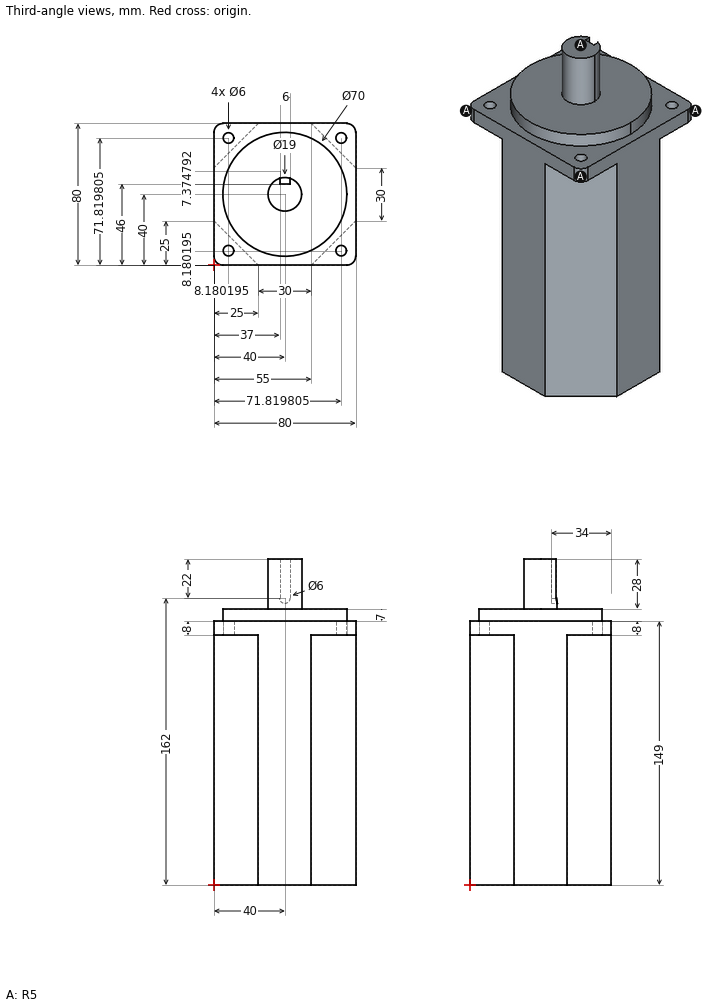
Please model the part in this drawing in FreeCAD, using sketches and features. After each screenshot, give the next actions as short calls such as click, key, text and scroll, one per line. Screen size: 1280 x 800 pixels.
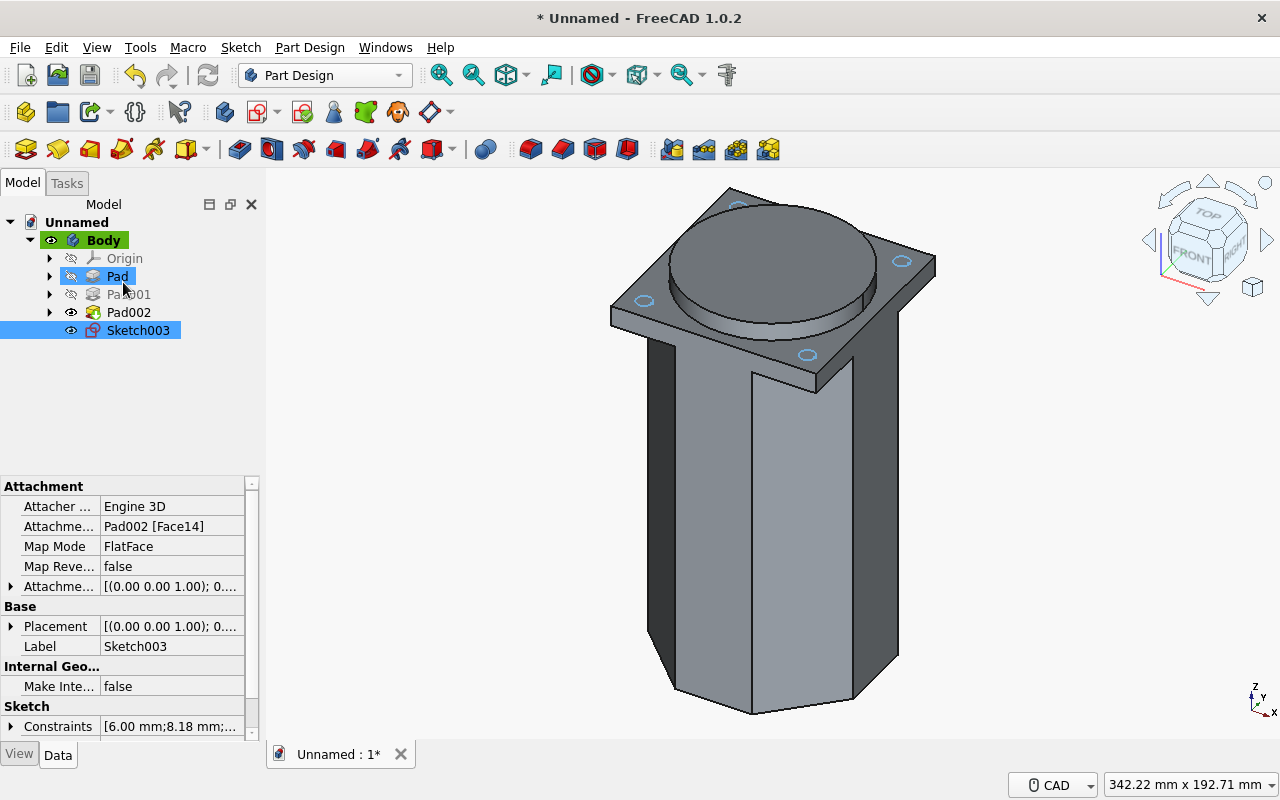
click(240, 150)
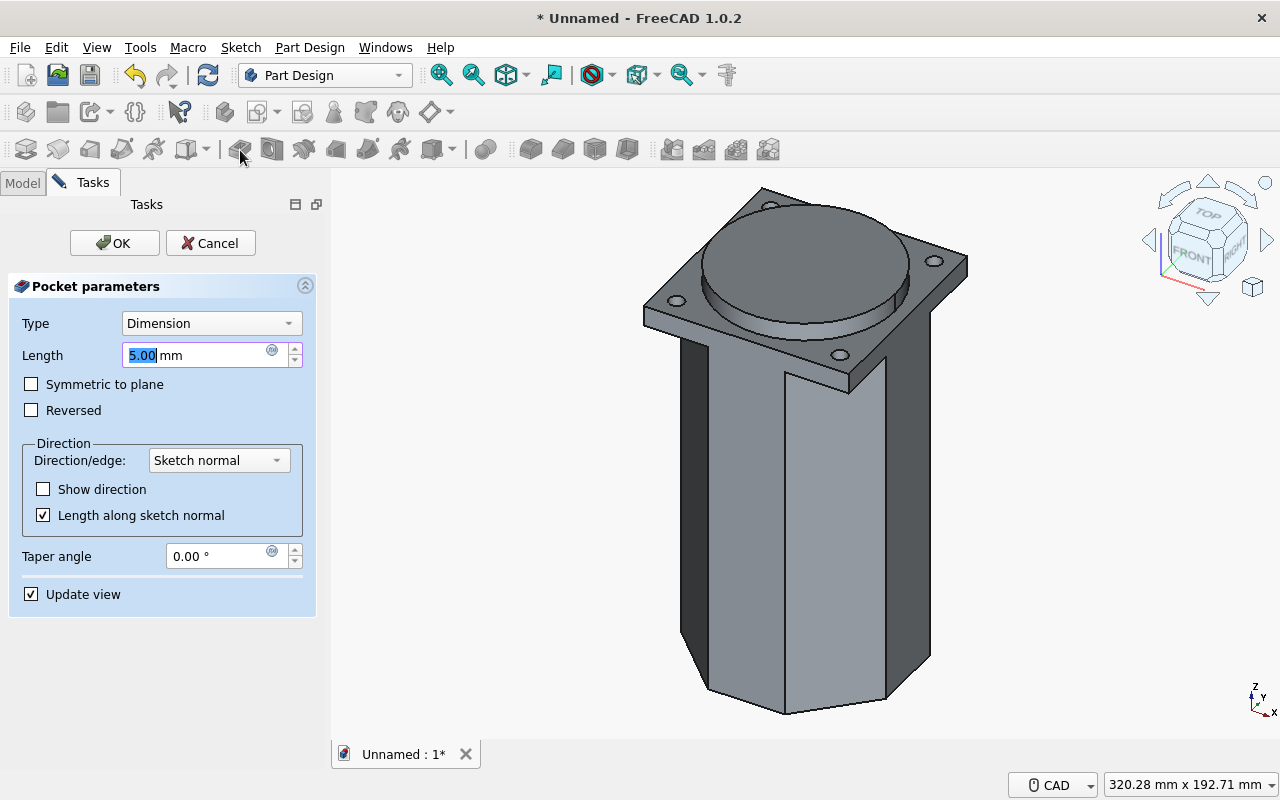
text(8)
key(Tab)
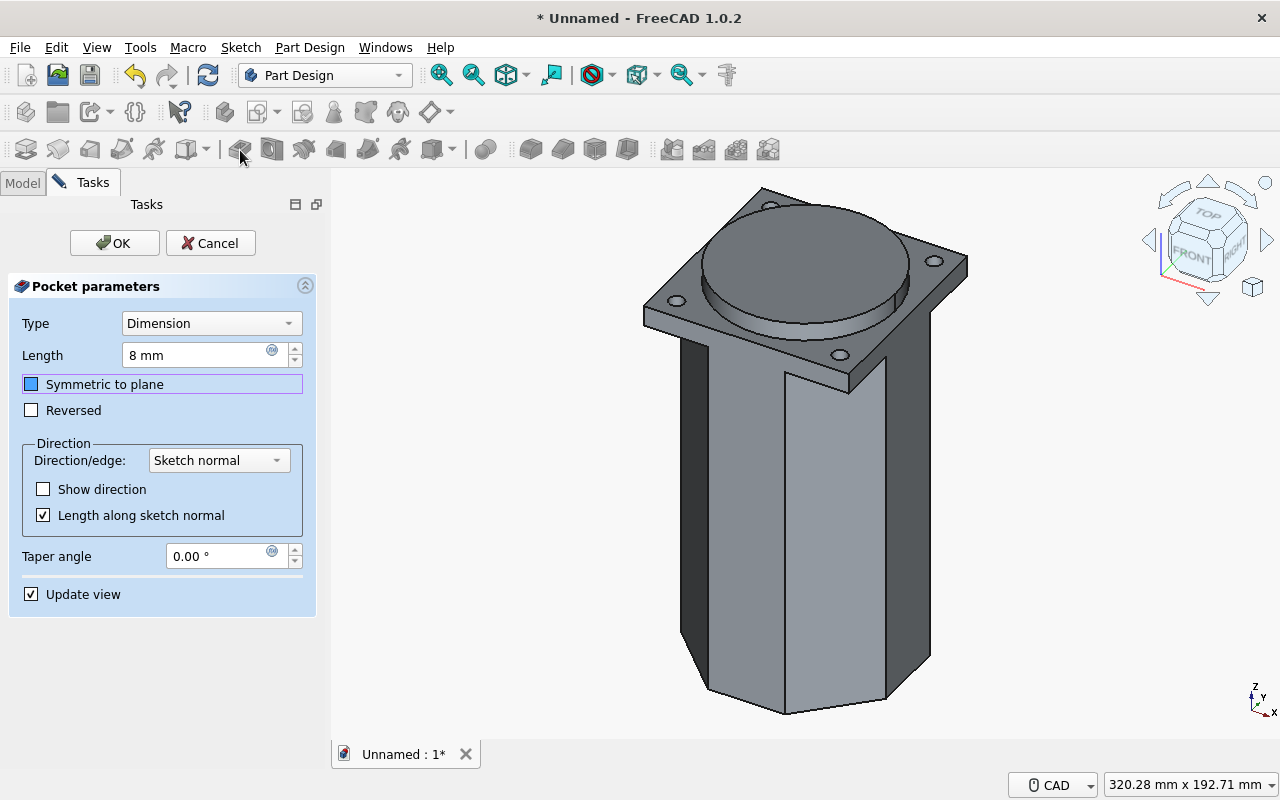
click(115, 243)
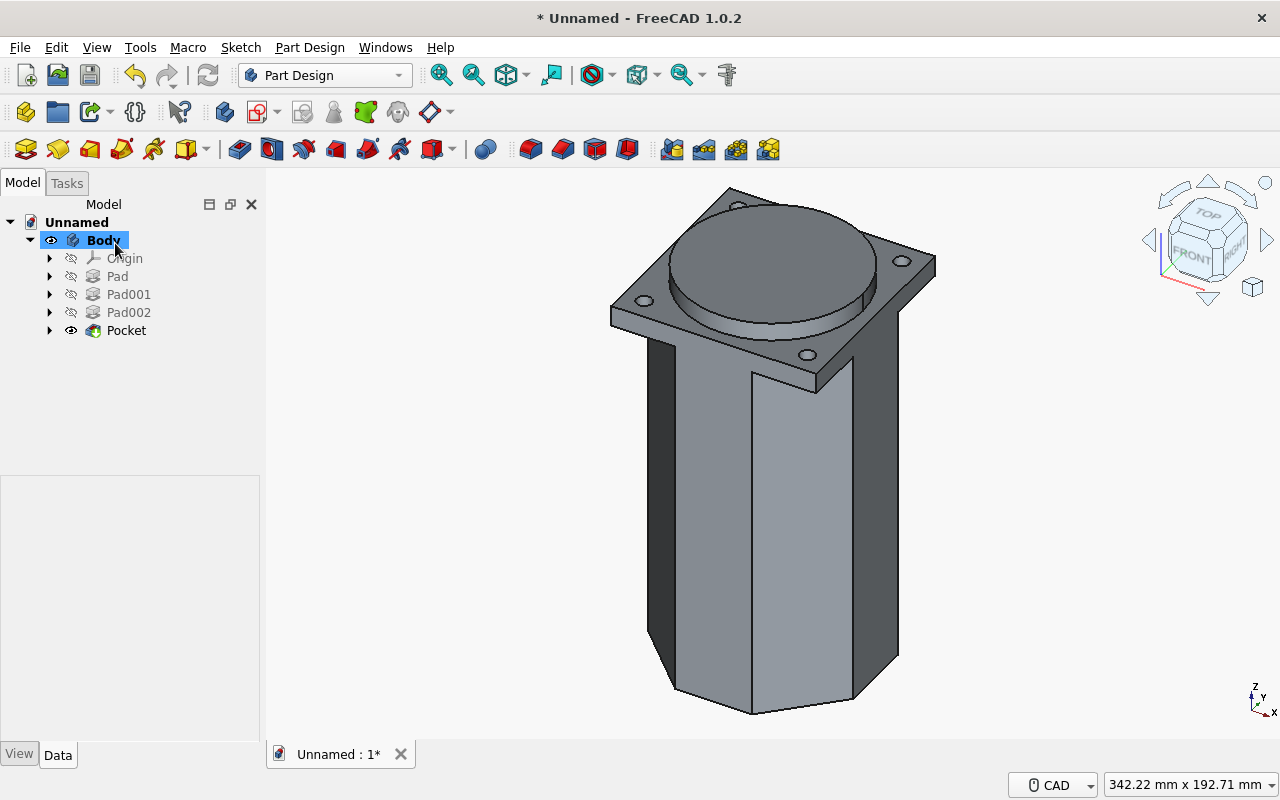
click(816, 383)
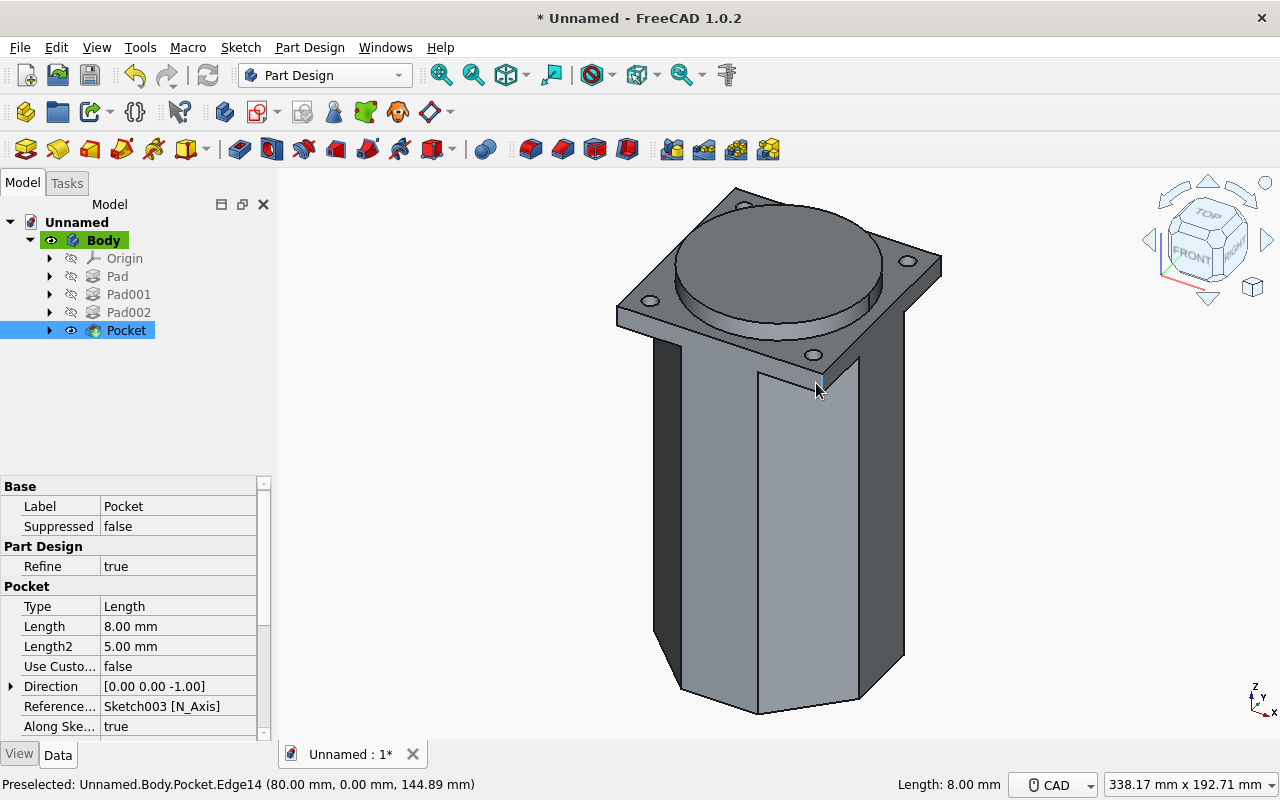
key(0)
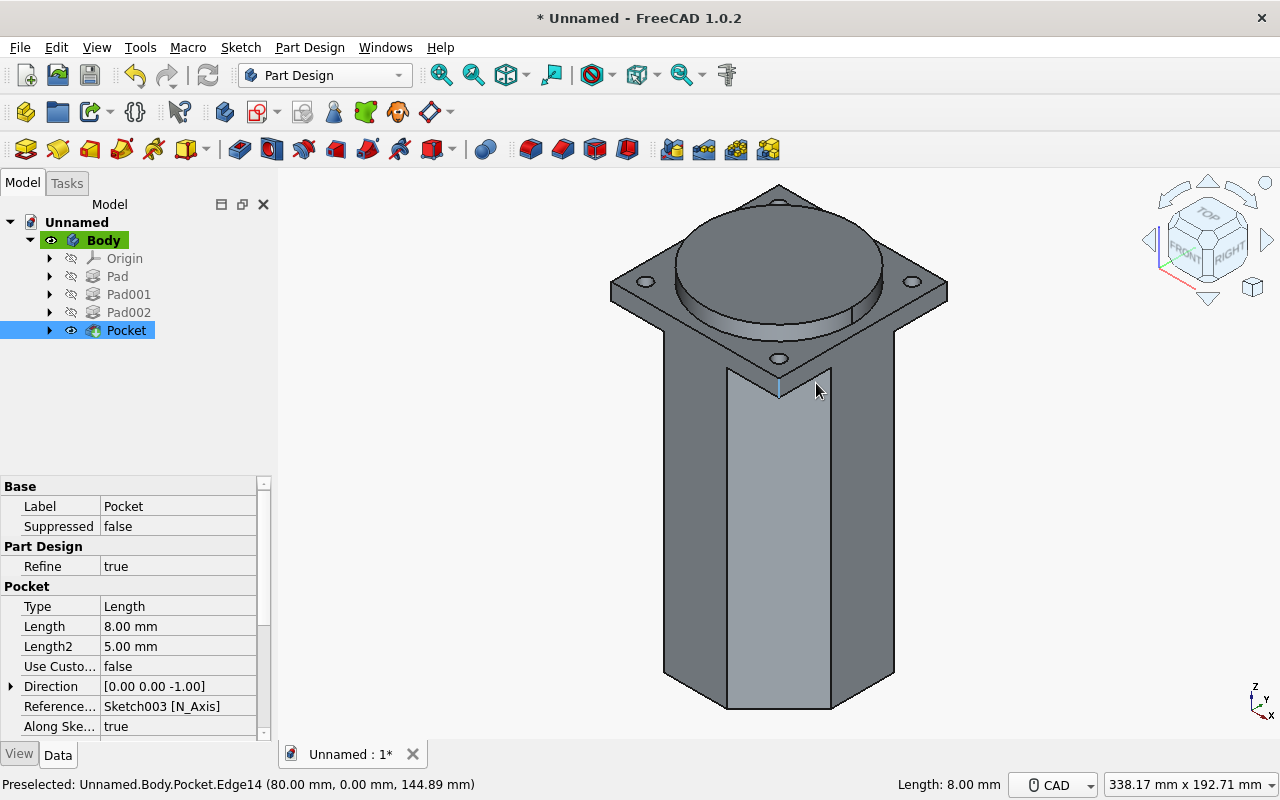
key(v)
key(f)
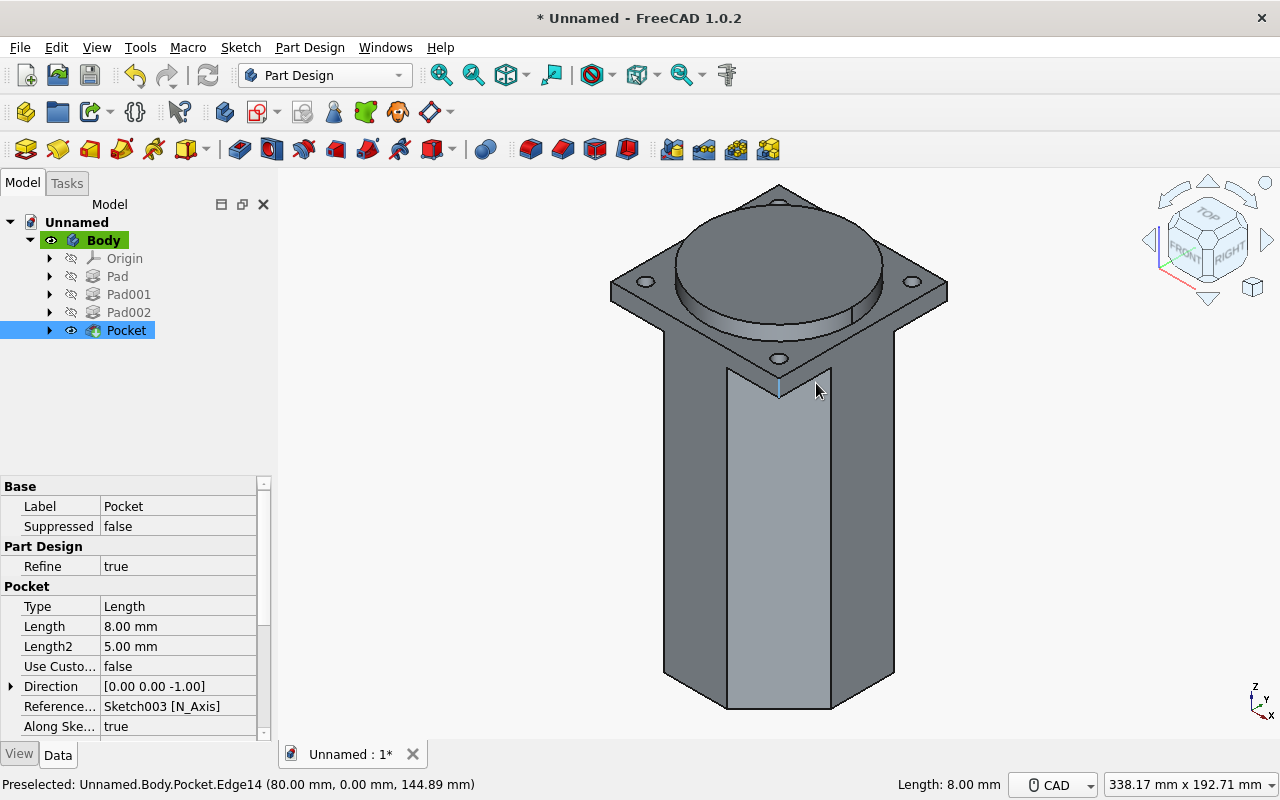
key(2)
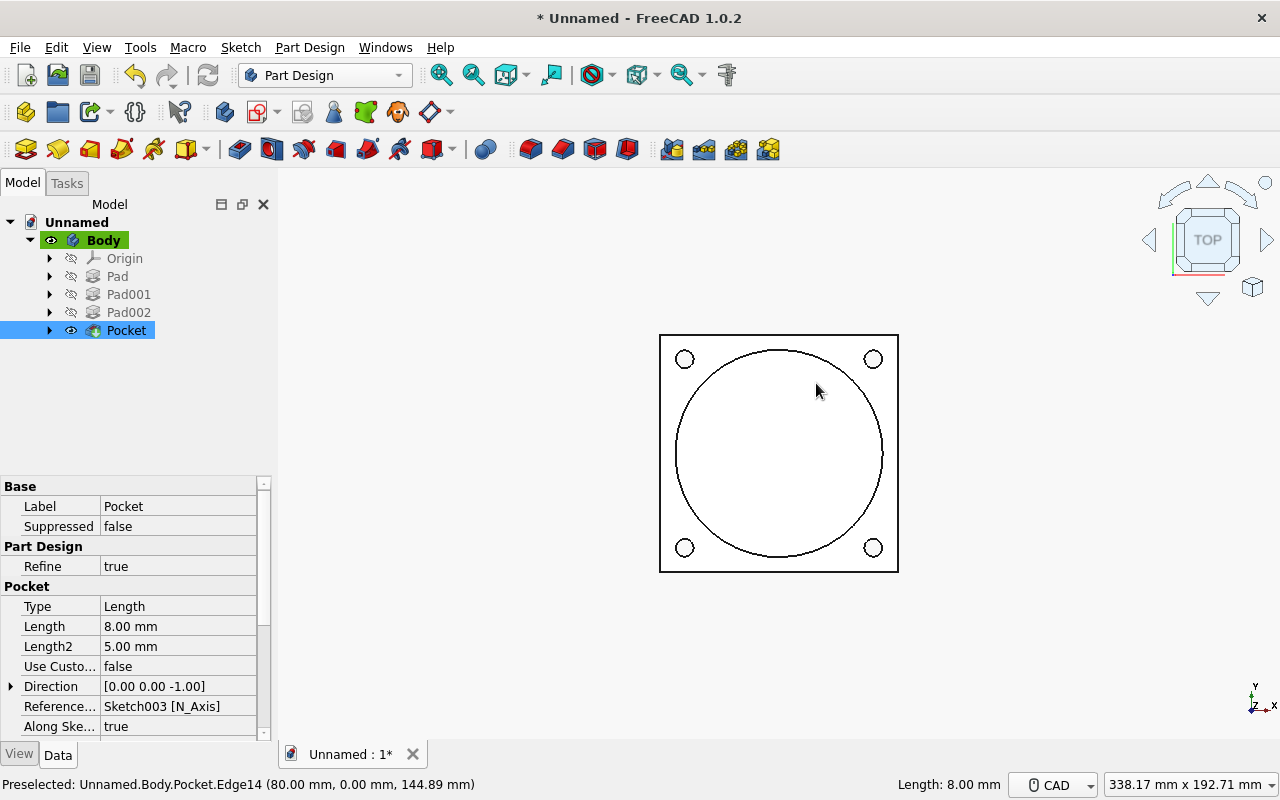
key(v)
key(f)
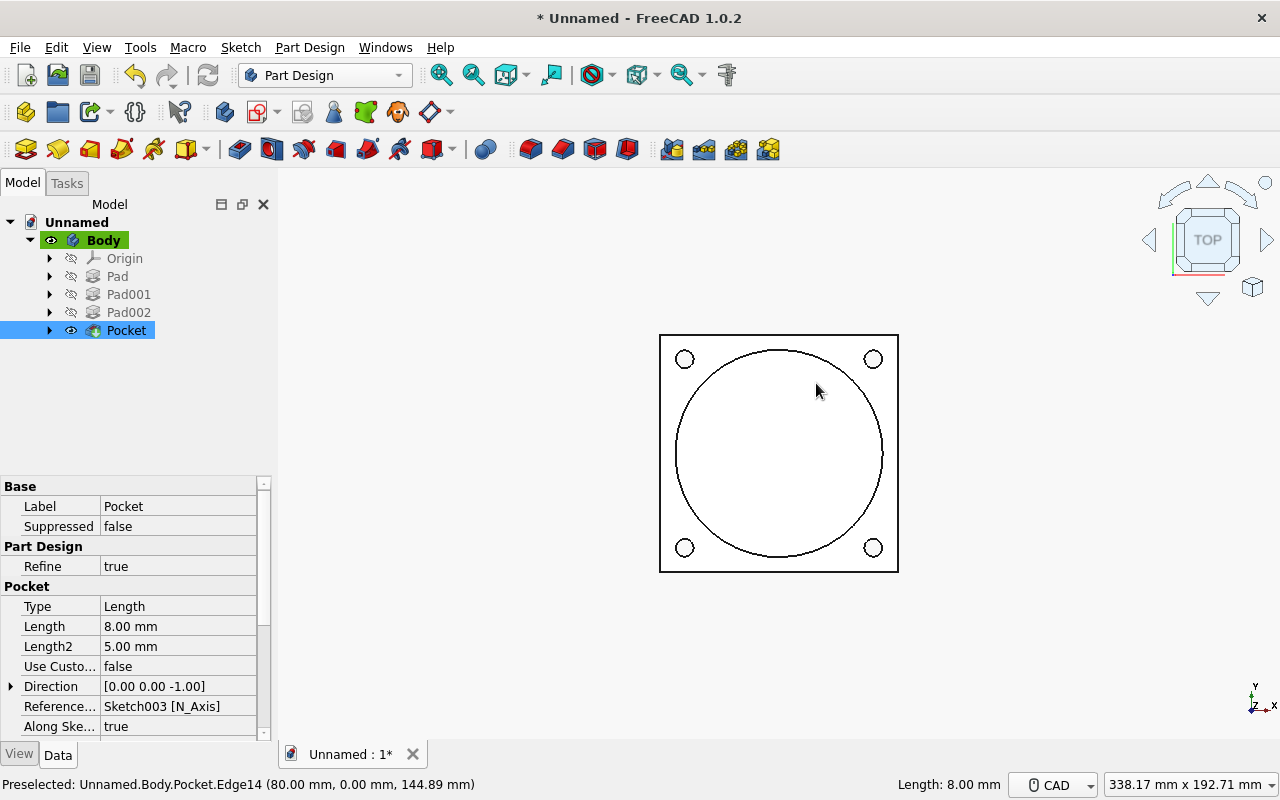
key(1)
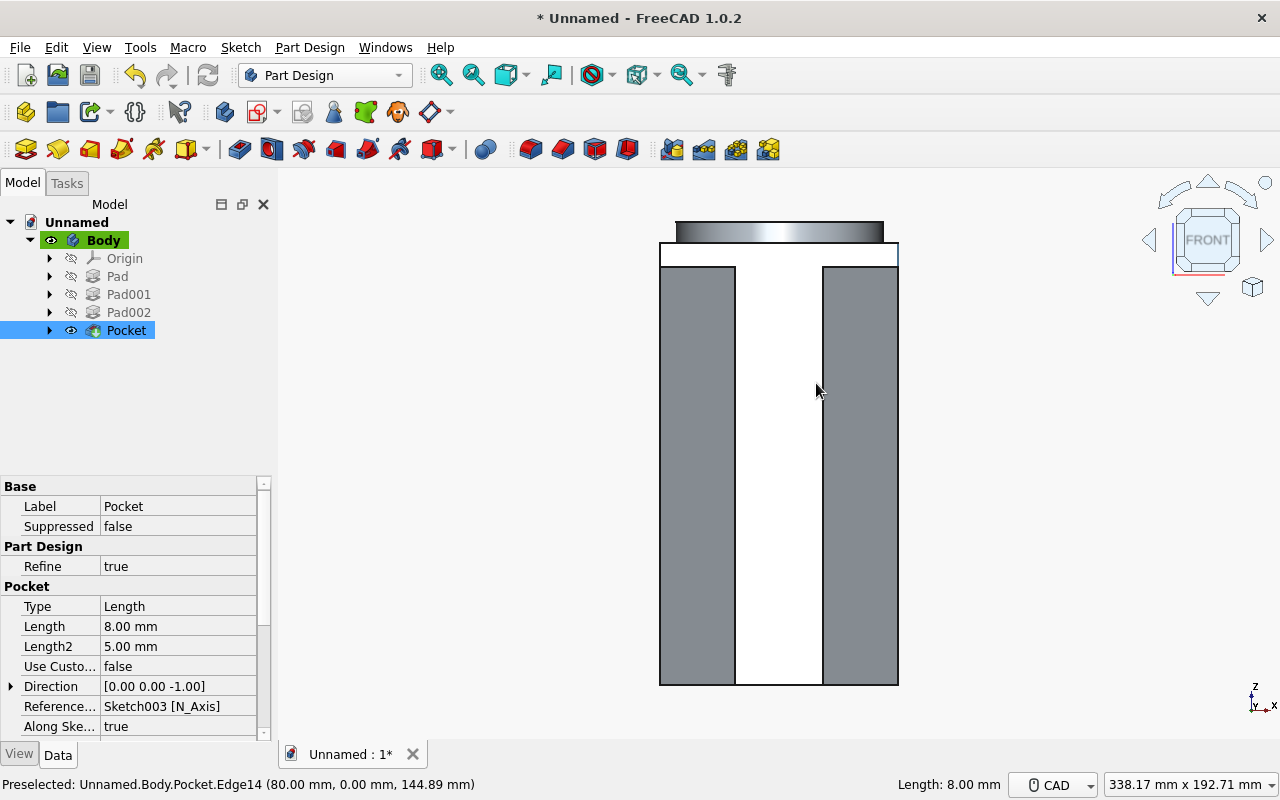
click(660, 254, ctrl)